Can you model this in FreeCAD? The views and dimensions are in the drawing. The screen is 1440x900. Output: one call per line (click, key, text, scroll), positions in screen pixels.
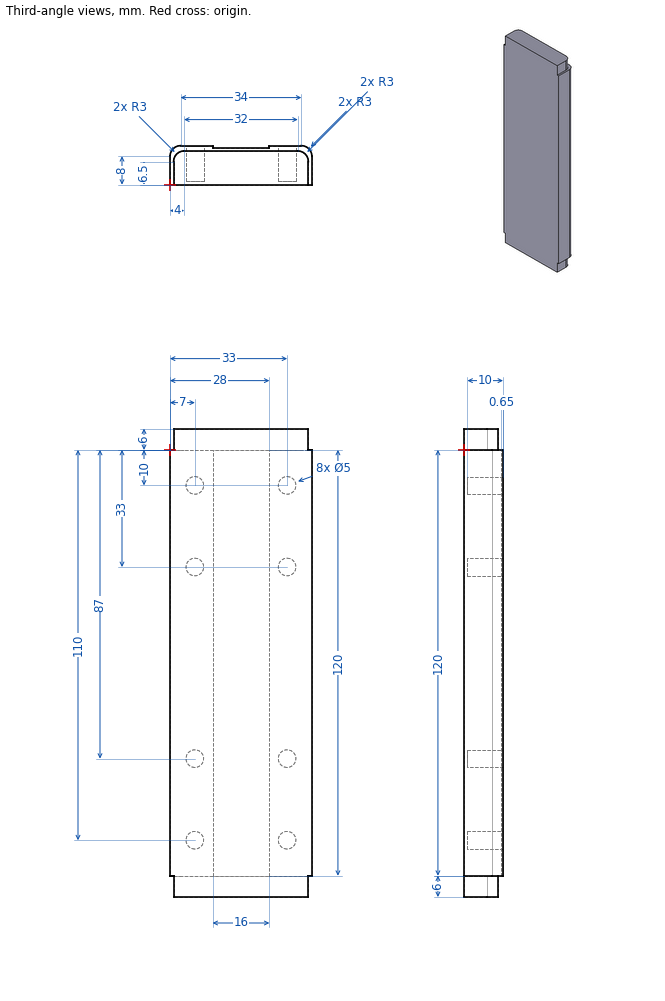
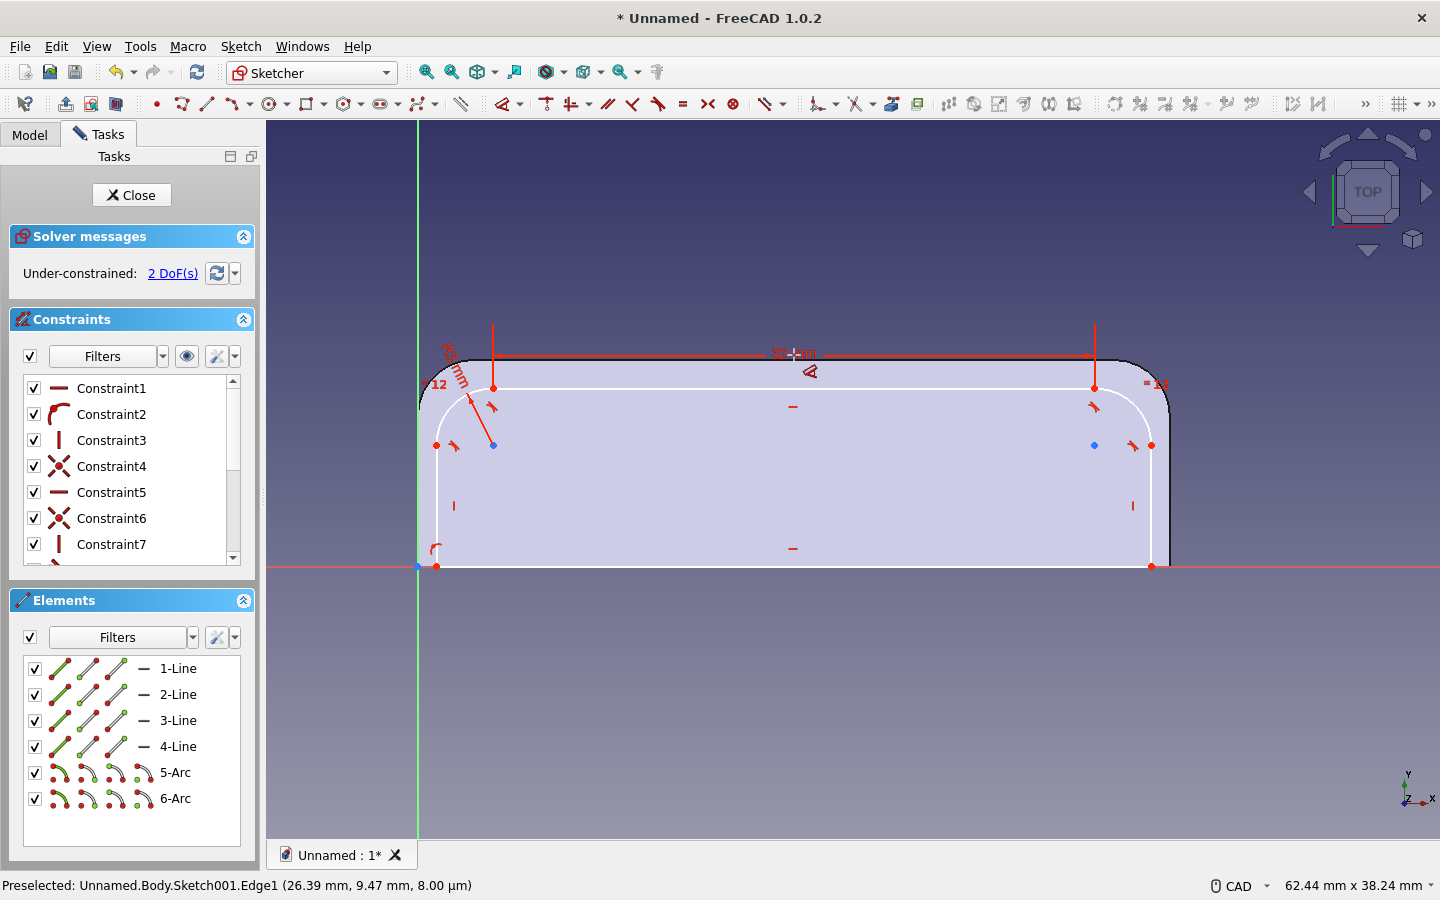
click(493, 389)
click(455, 601)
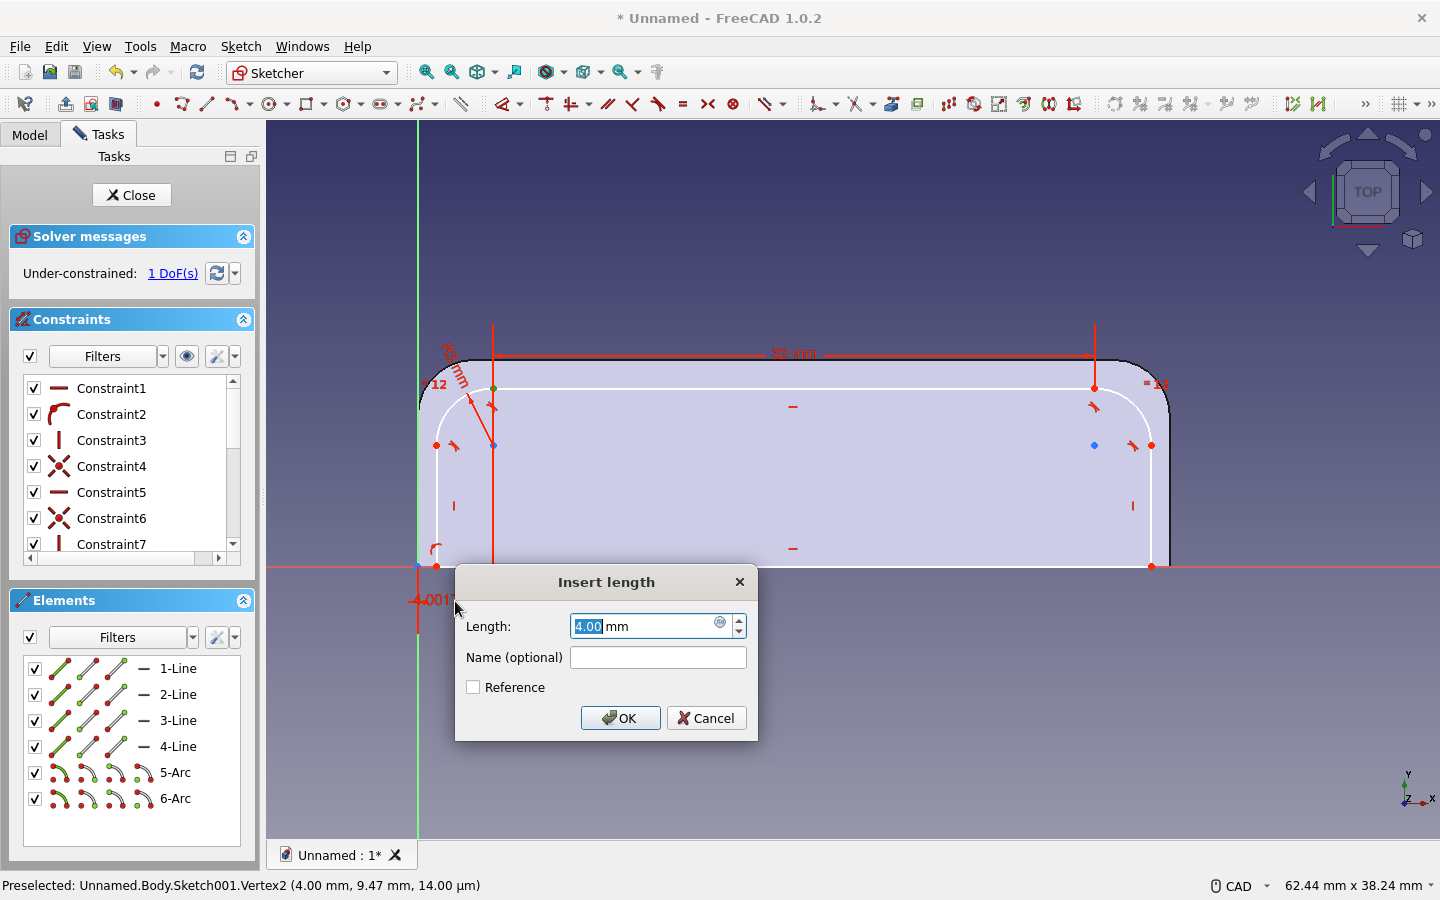
text(4)
key(Return)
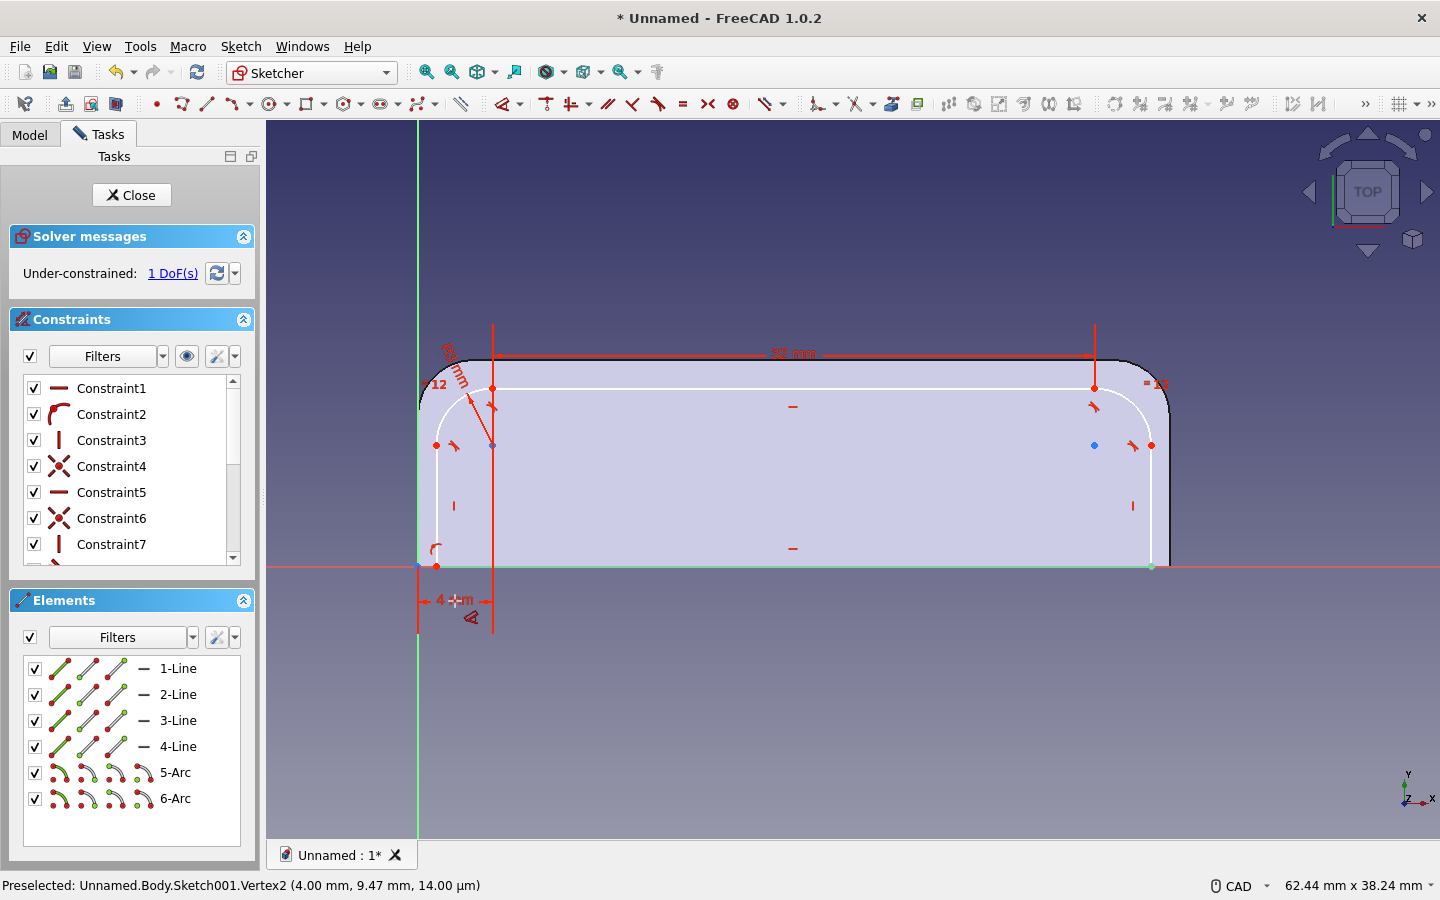
click(437, 482)
click(403, 506)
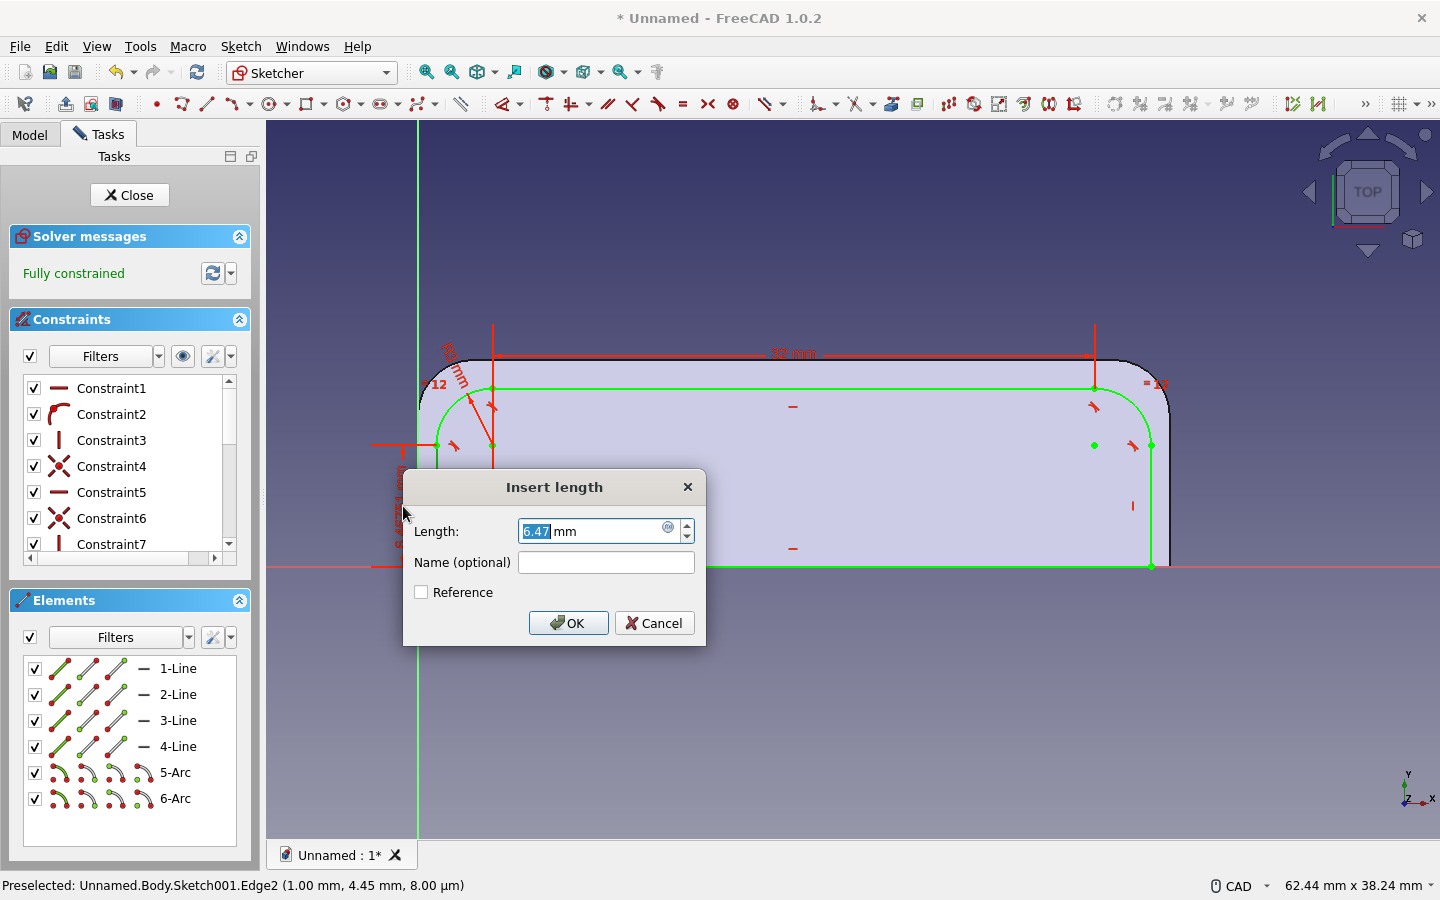
text(6.5)
key(Return)
key(Escape)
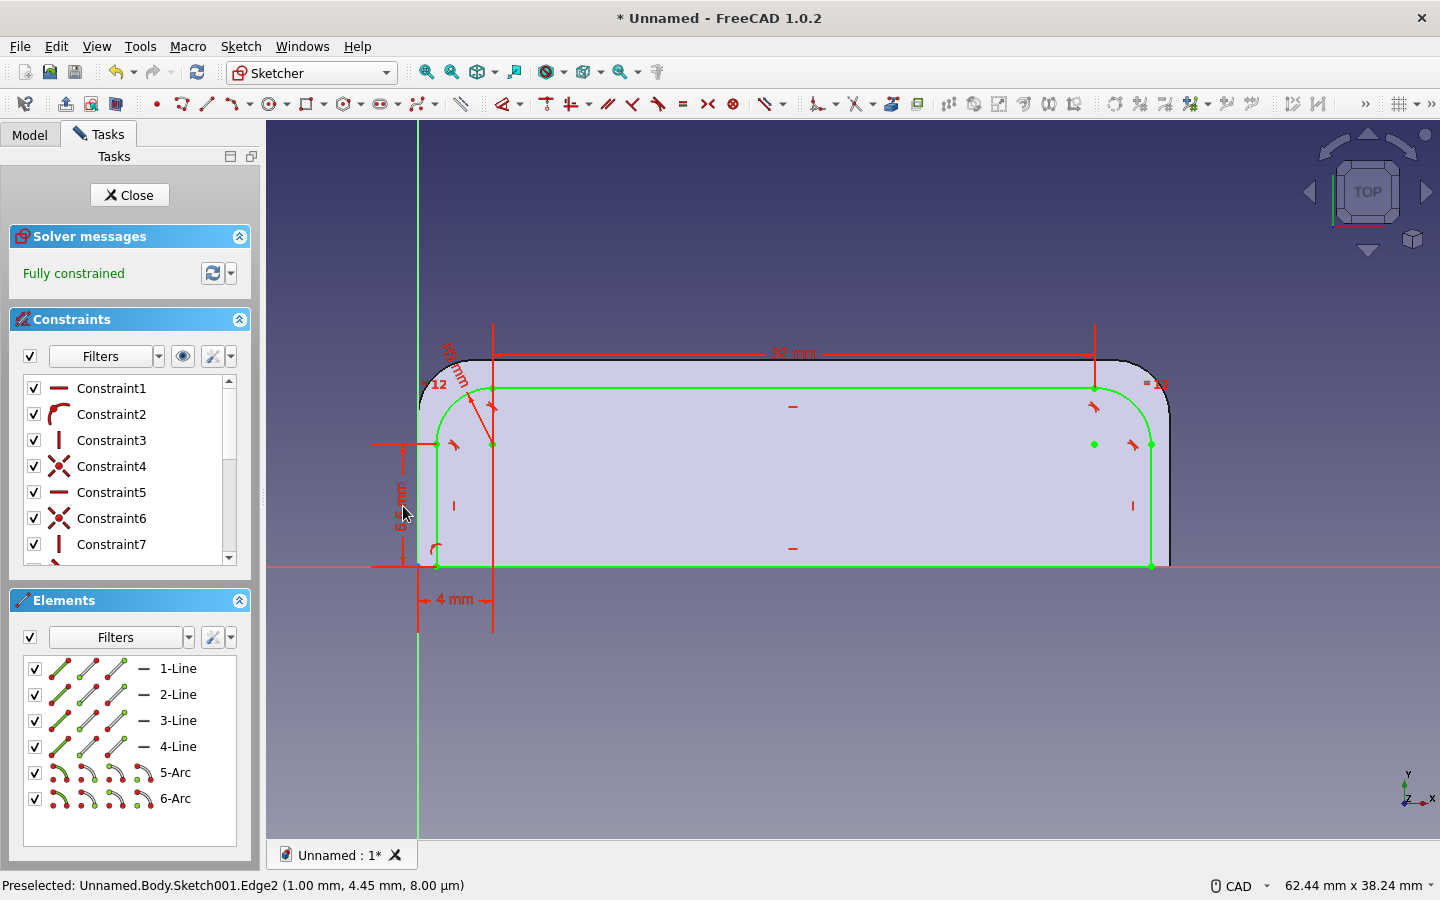
click(130, 195)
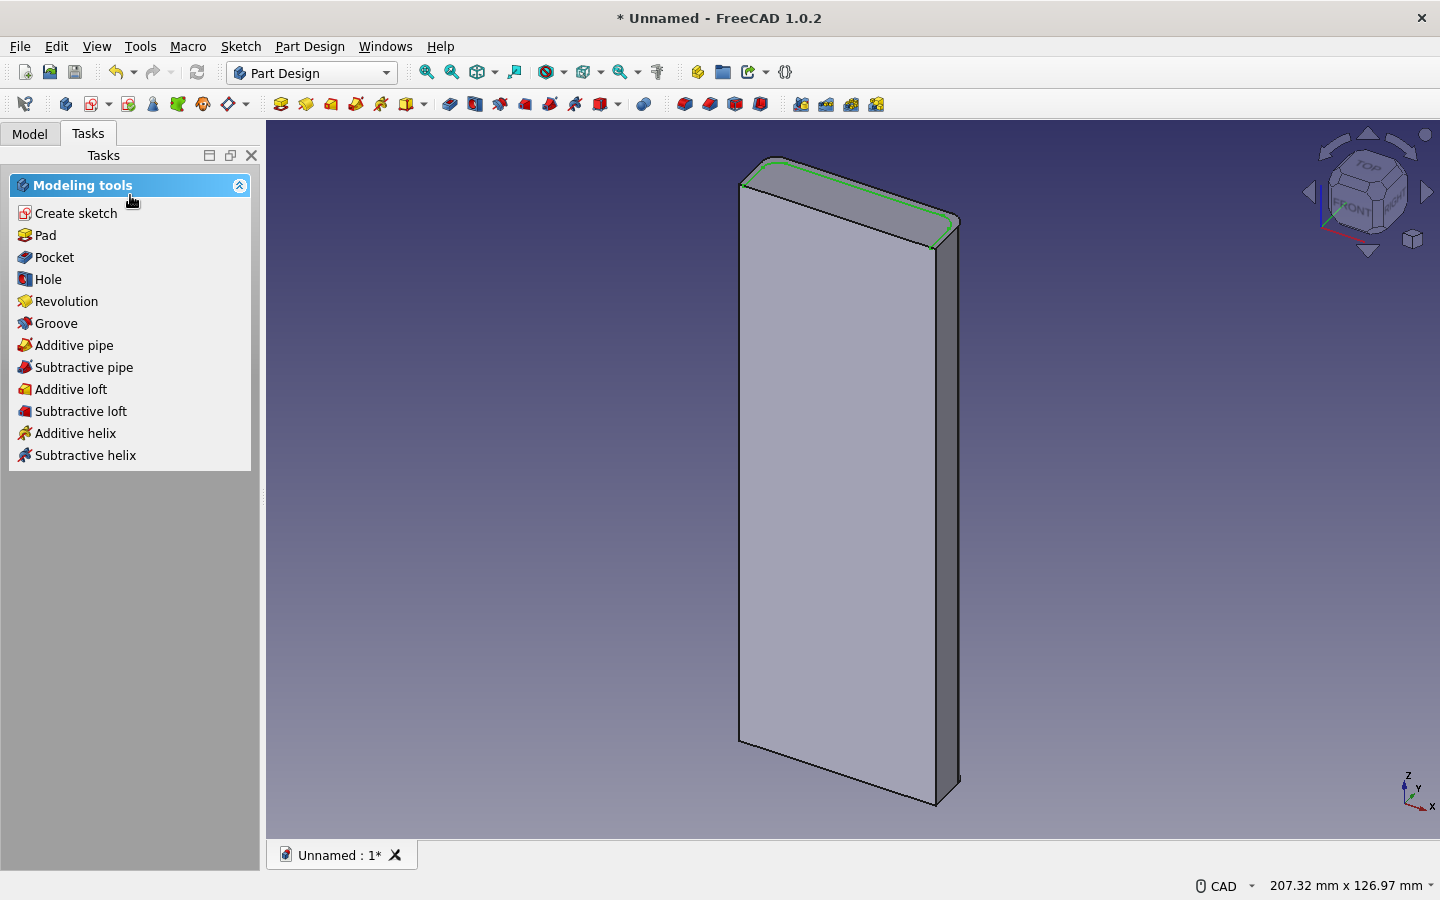
click(281, 104)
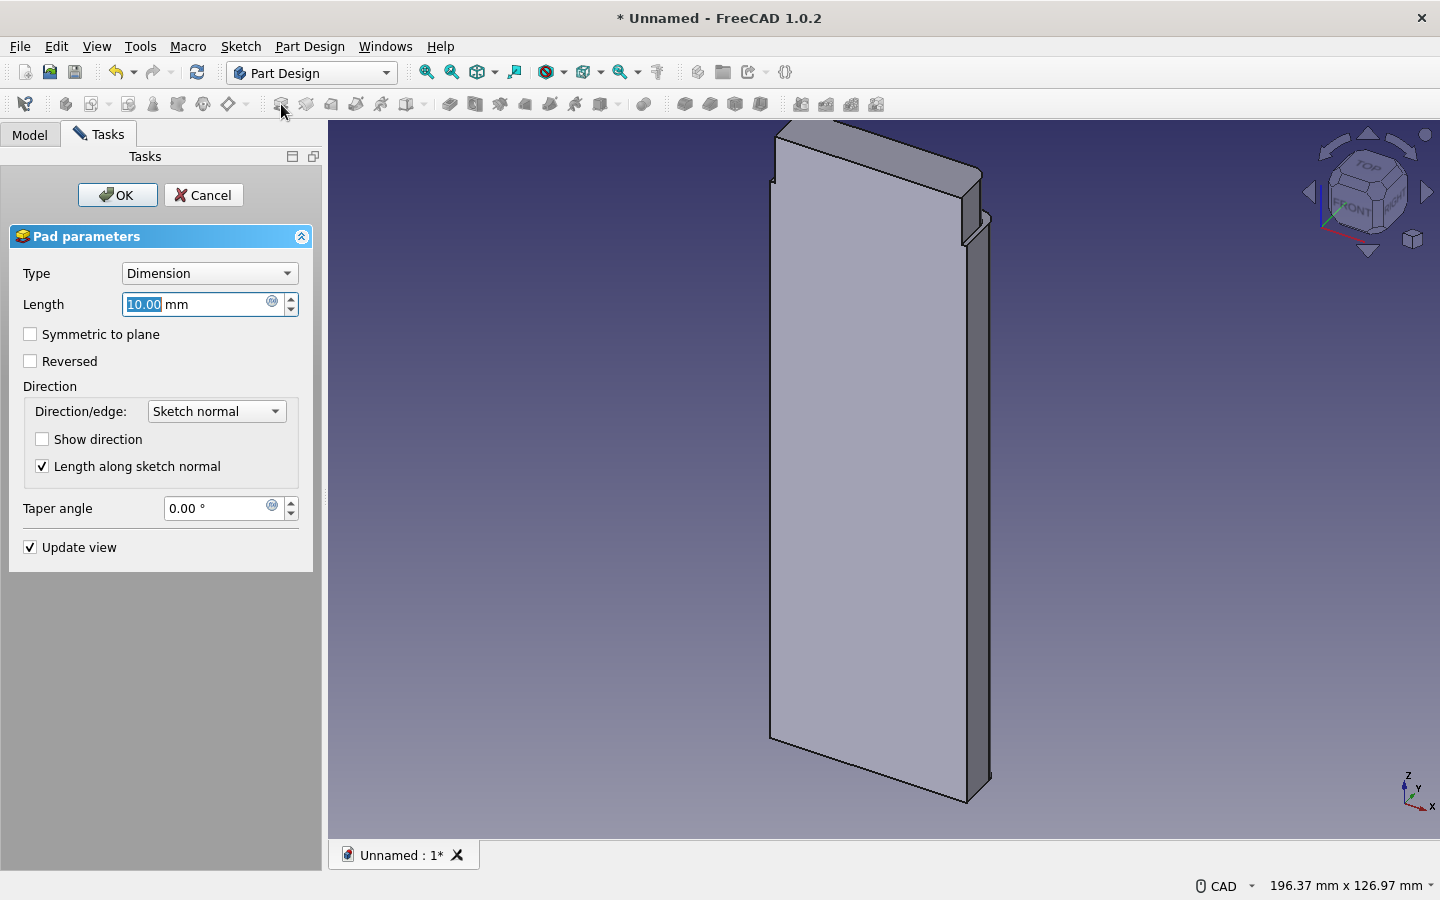
text(6)
key(Tab)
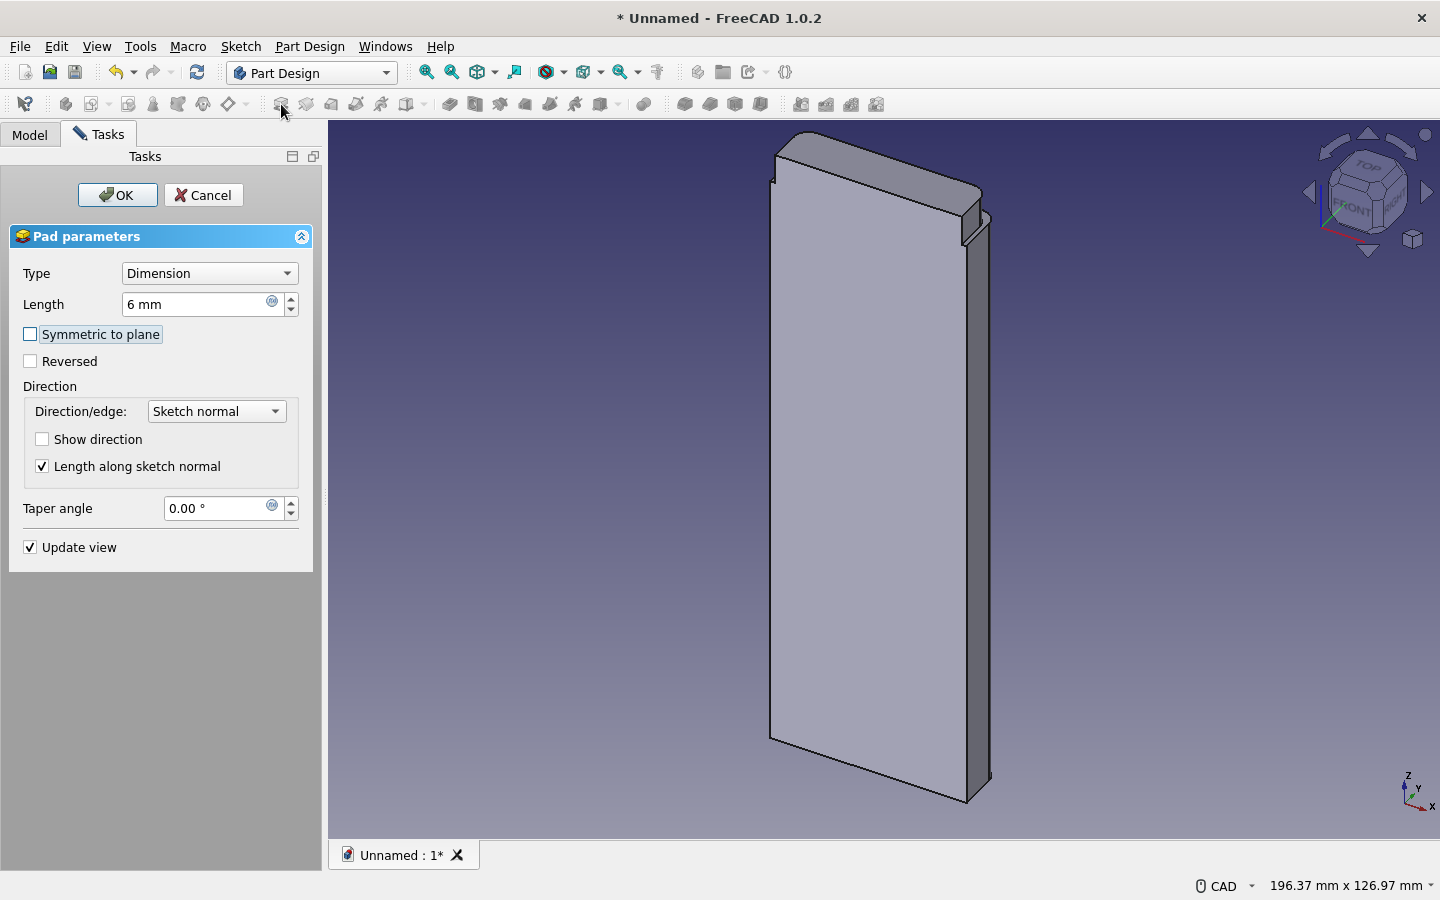
click(118, 195)